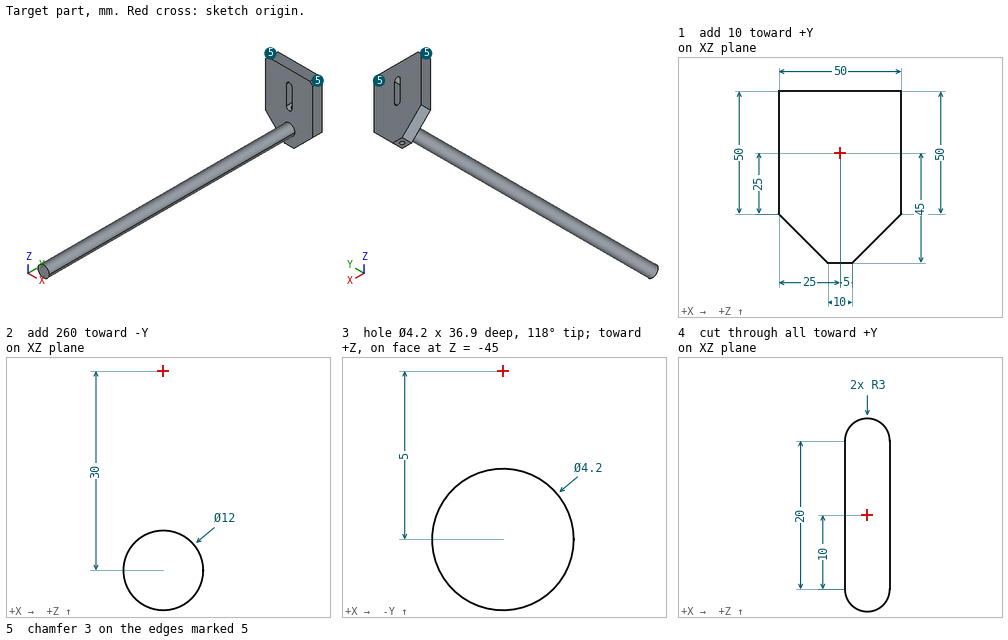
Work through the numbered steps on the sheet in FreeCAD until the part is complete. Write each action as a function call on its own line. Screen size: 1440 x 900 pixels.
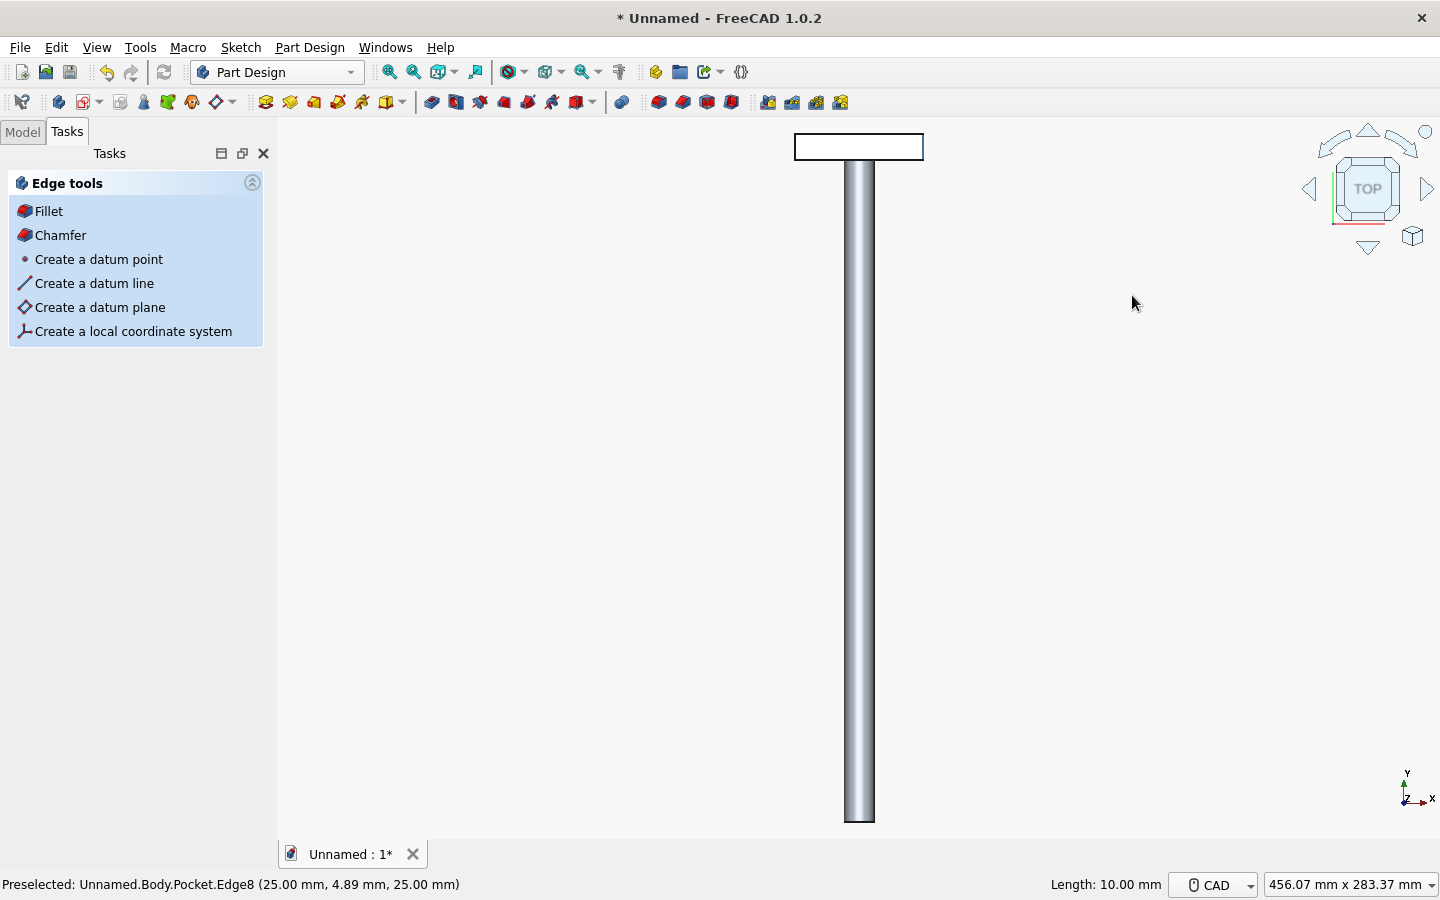
click(795, 146, ctrl)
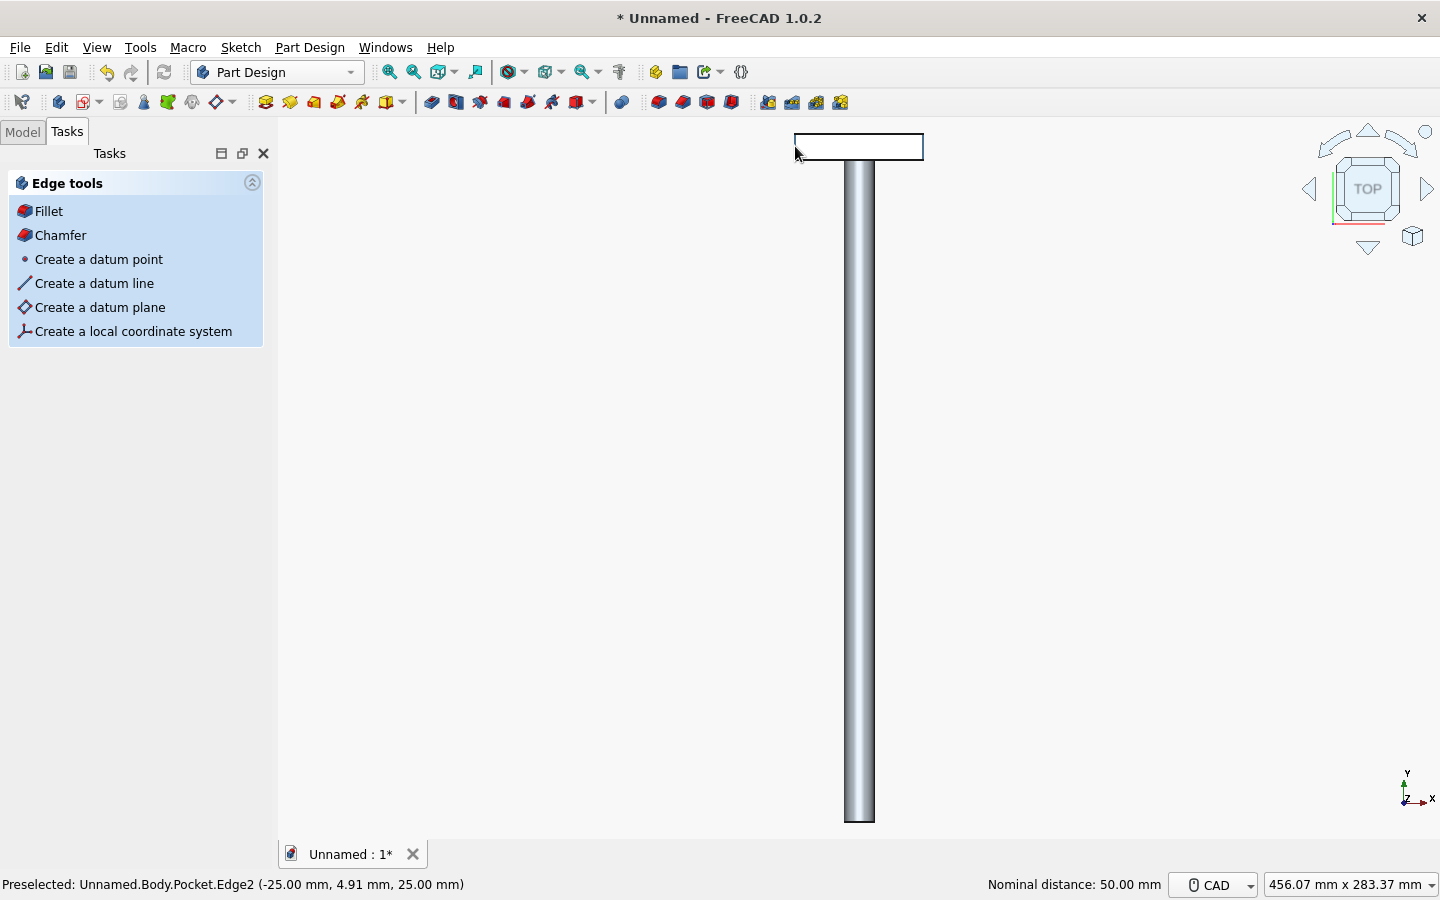
click(684, 102)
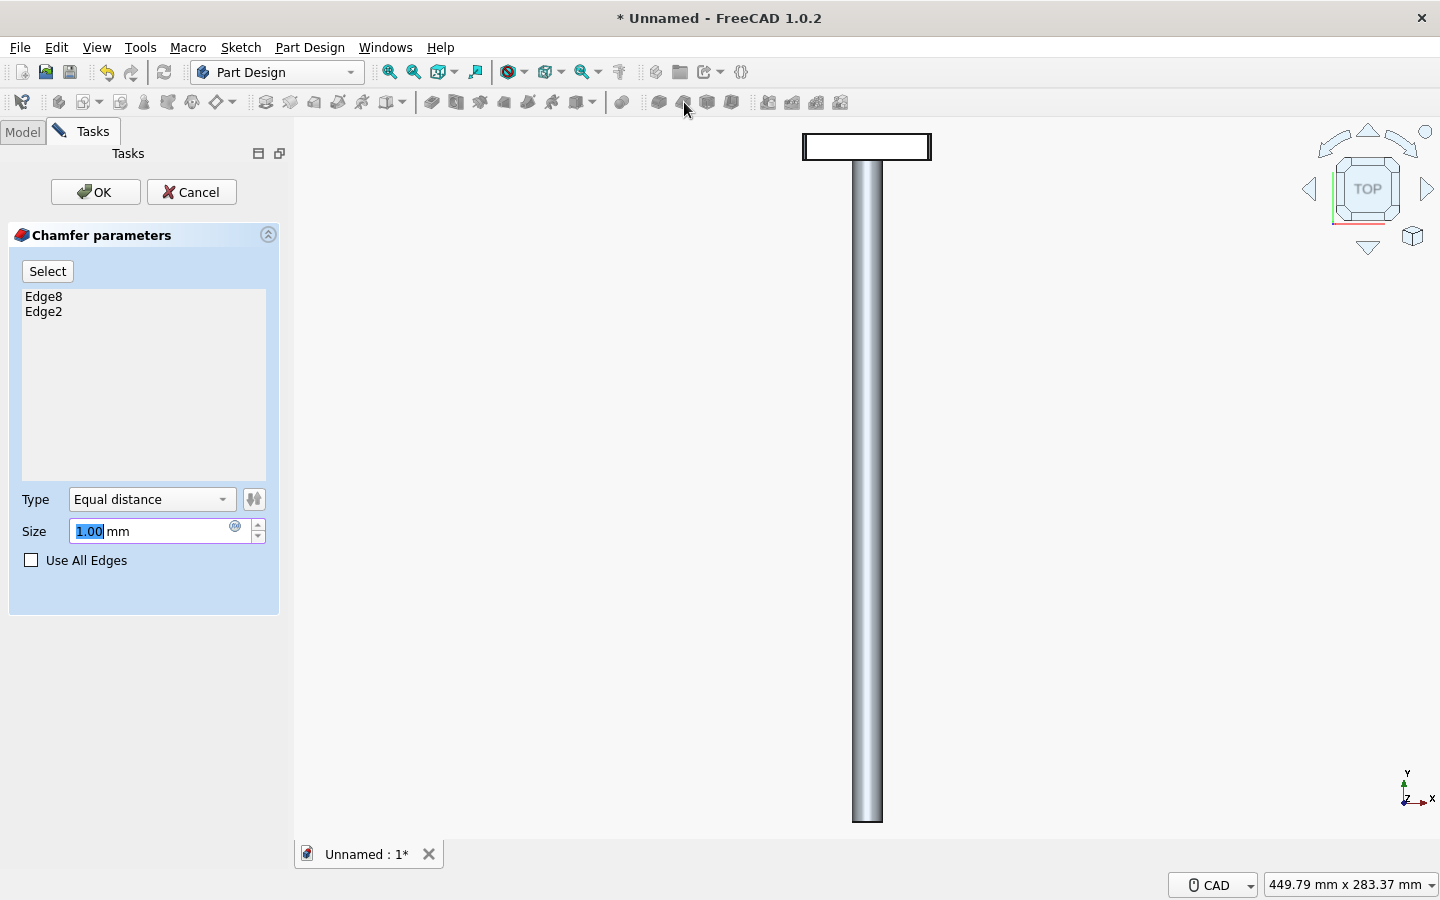
text(3)
key(Tab)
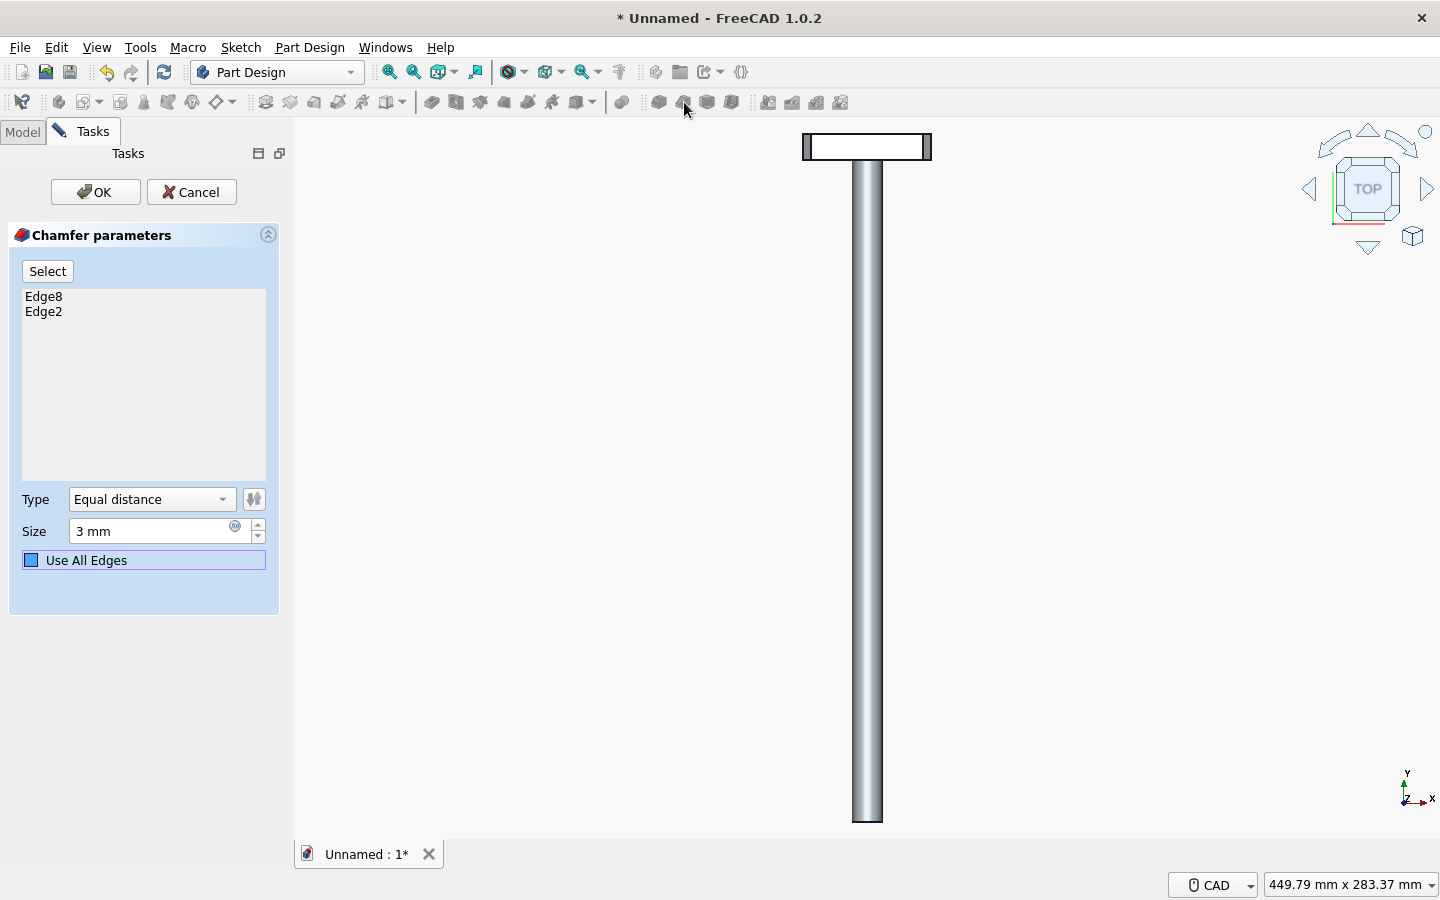
click(96, 192)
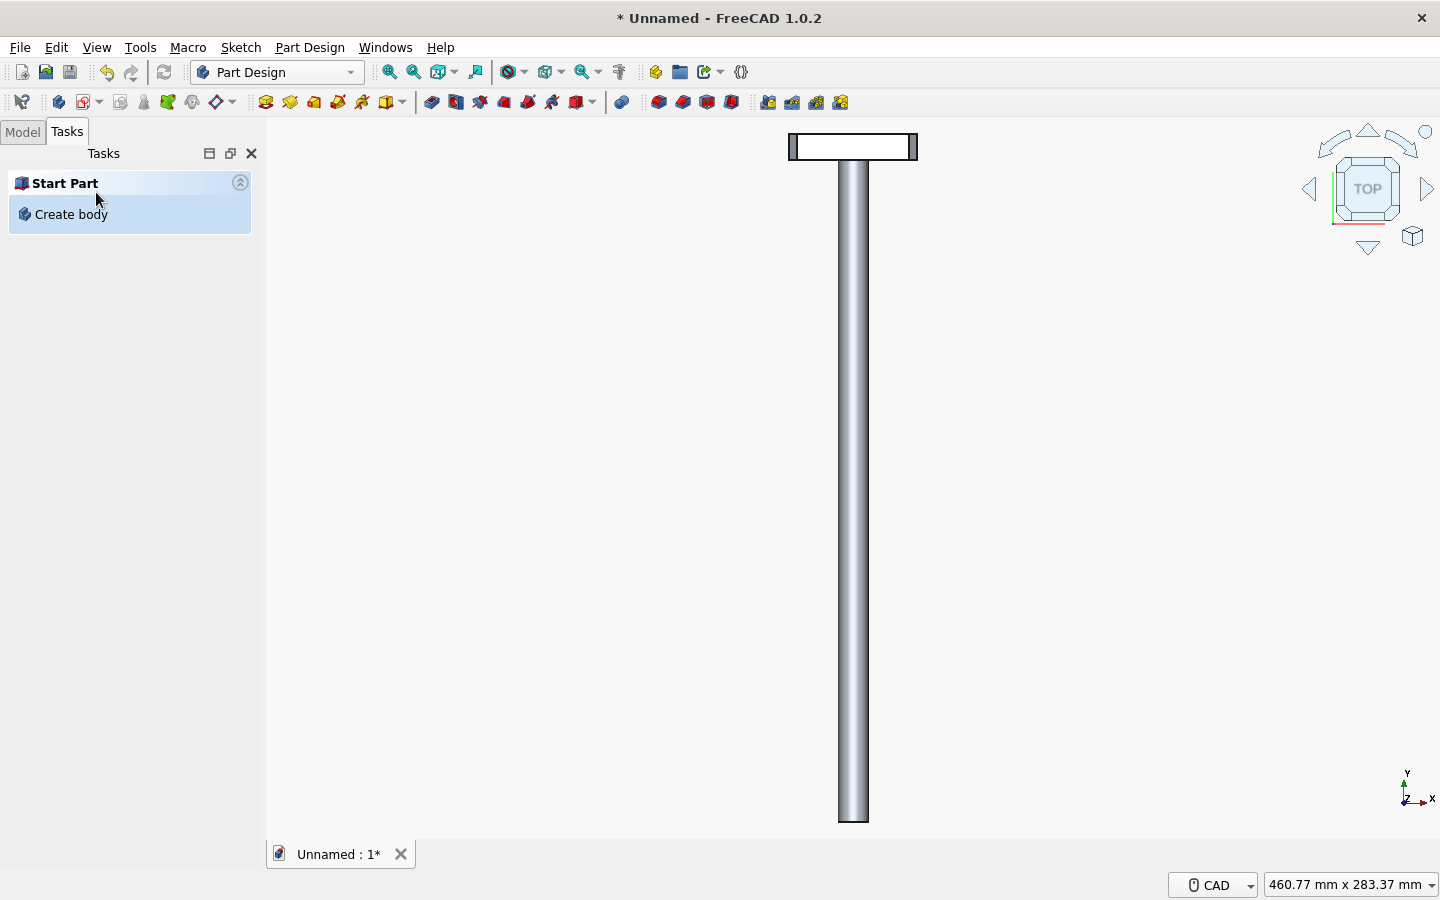
key(0)